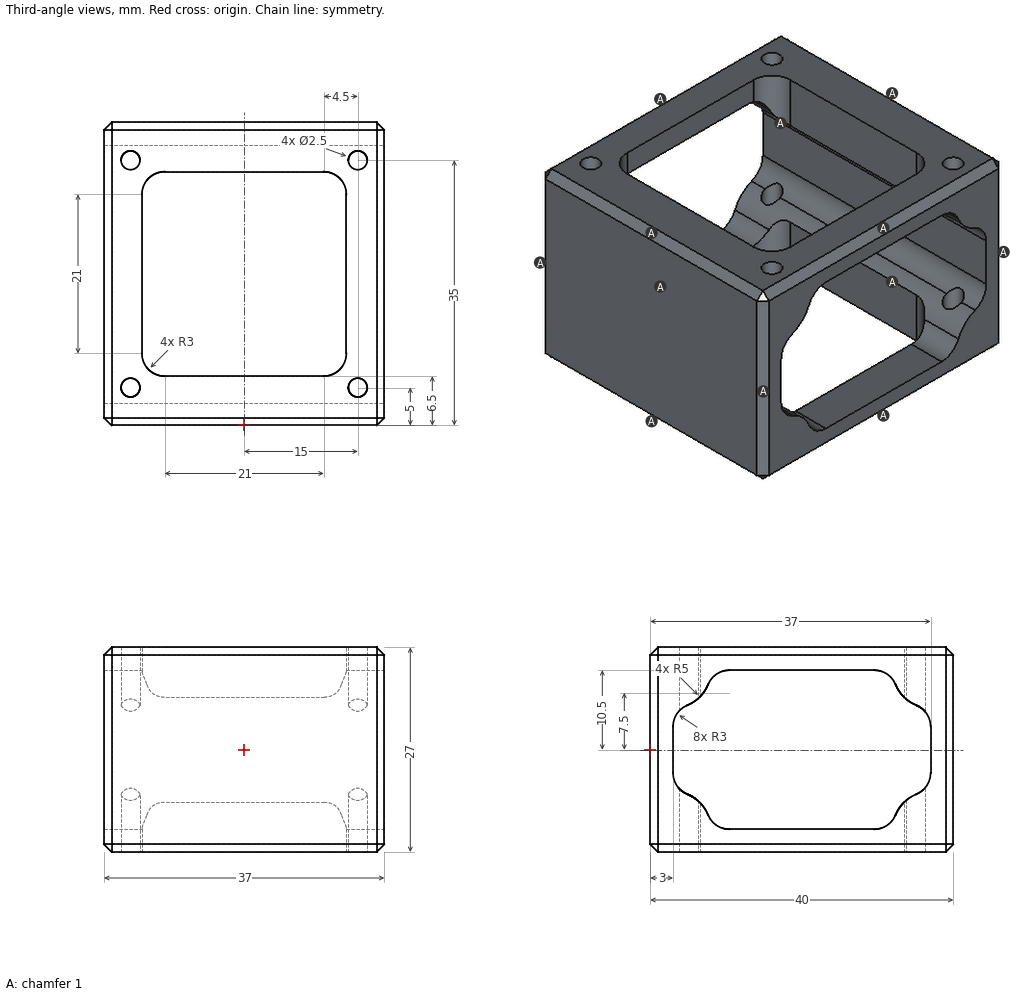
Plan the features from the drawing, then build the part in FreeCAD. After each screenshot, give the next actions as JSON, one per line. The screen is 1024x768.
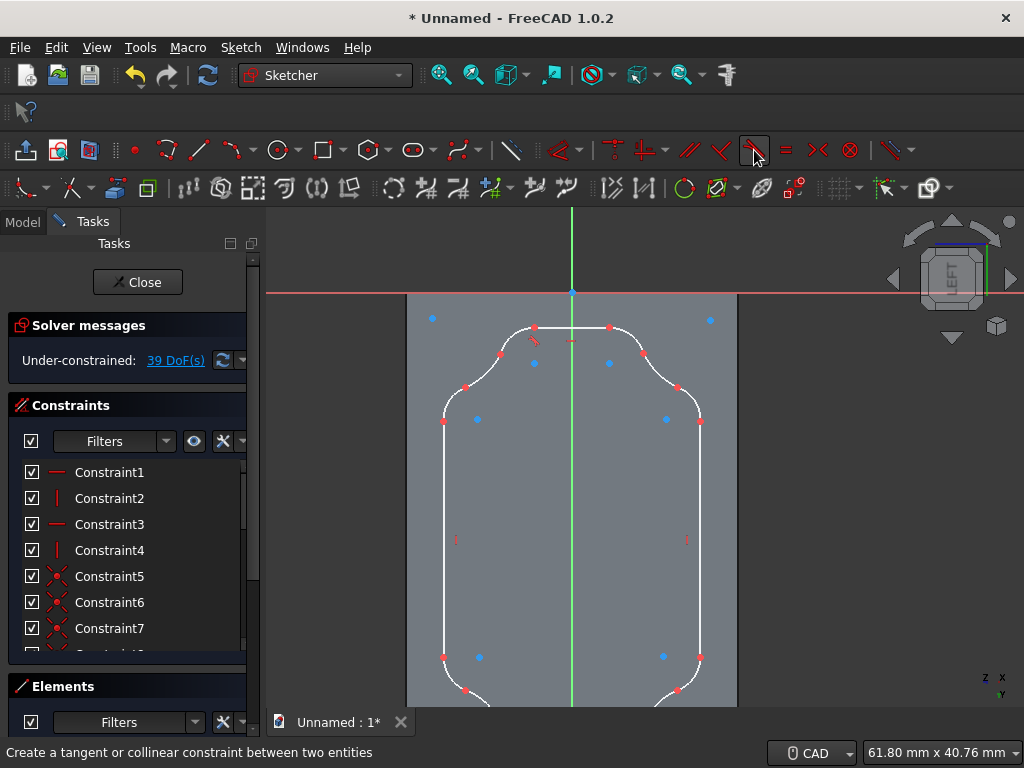
{"action": "left_click", "coordinate": [587, 328]}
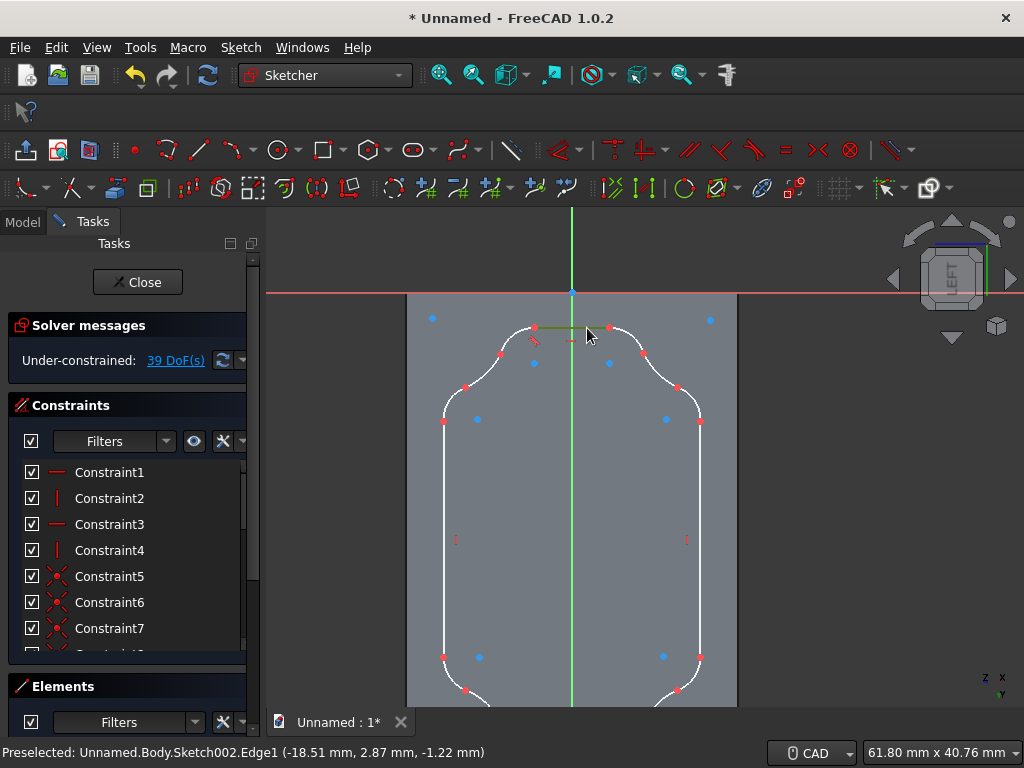
{"action": "left_click", "coordinate": [637, 341]}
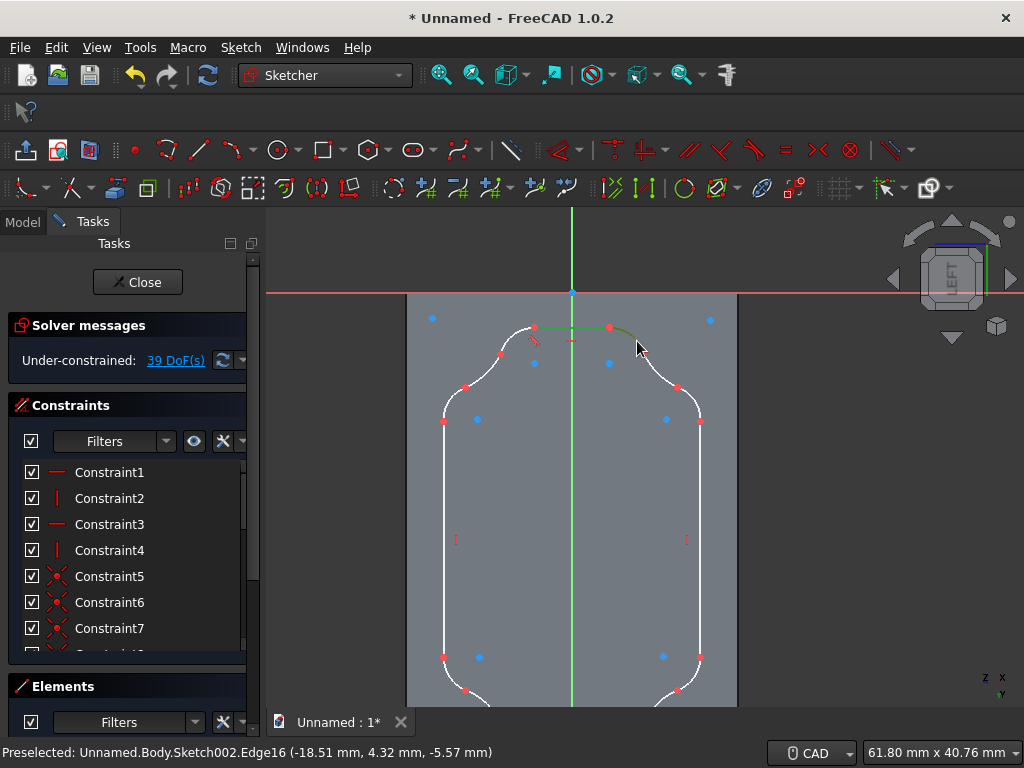
{"action": "key", "text": "t"}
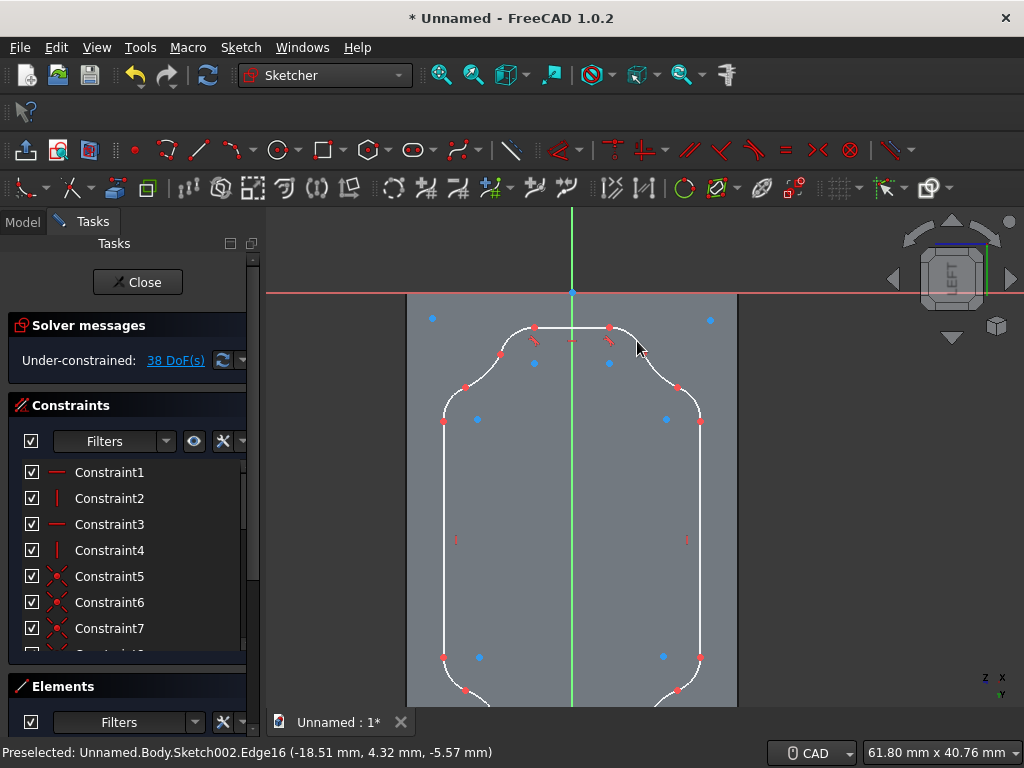
{"action": "left_click", "coordinate": [444, 492]}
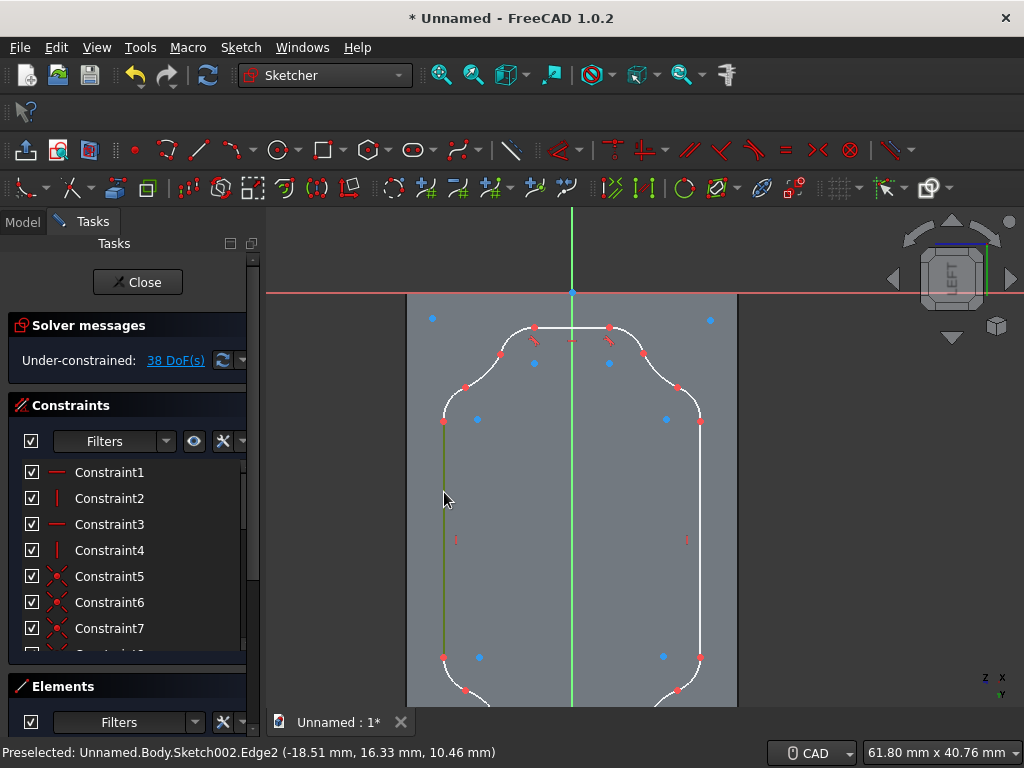
{"action": "left_click", "coordinate": [455, 394]}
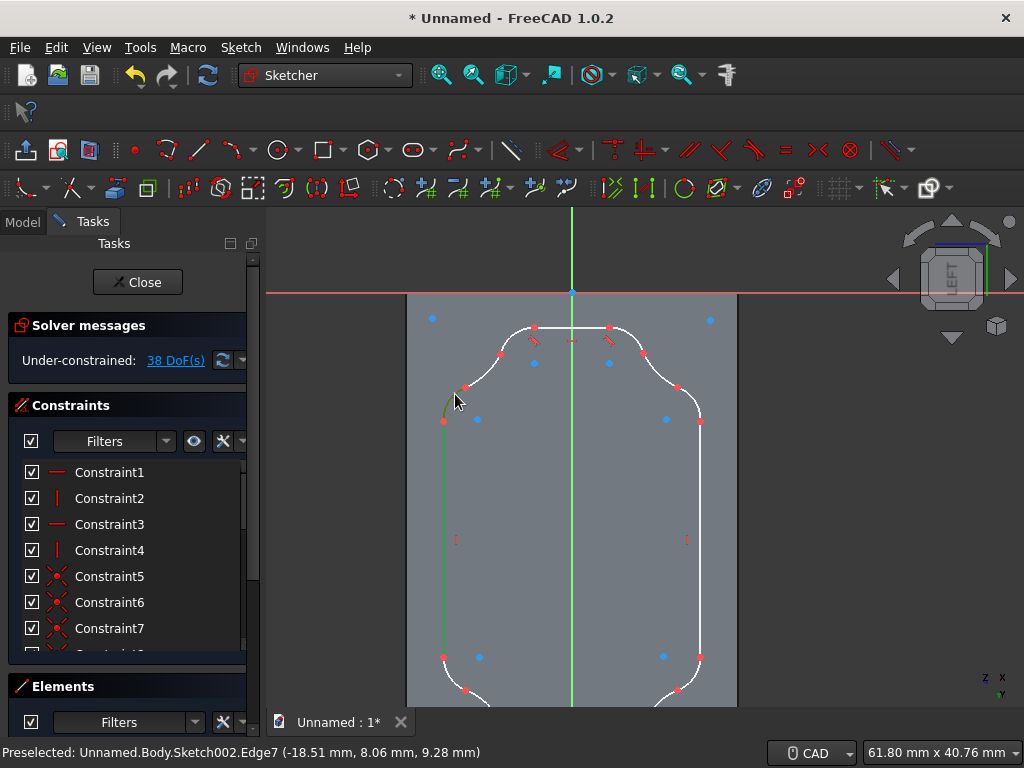
{"action": "key", "text": "t"}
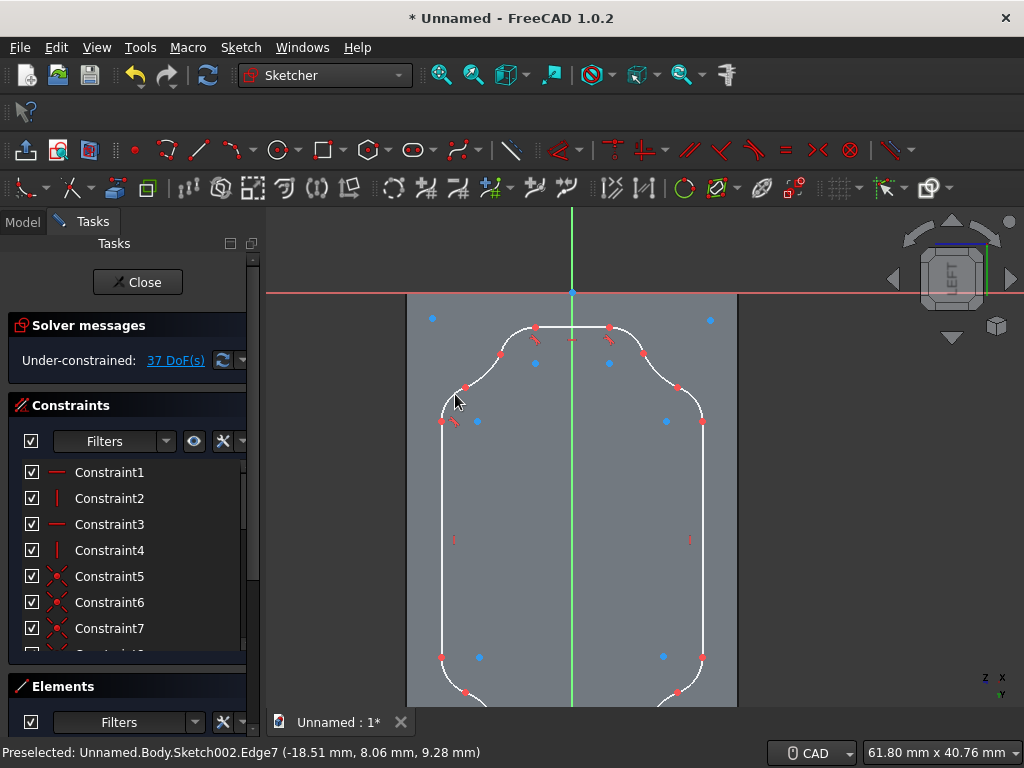
{"action": "left_click", "coordinate": [442, 492]}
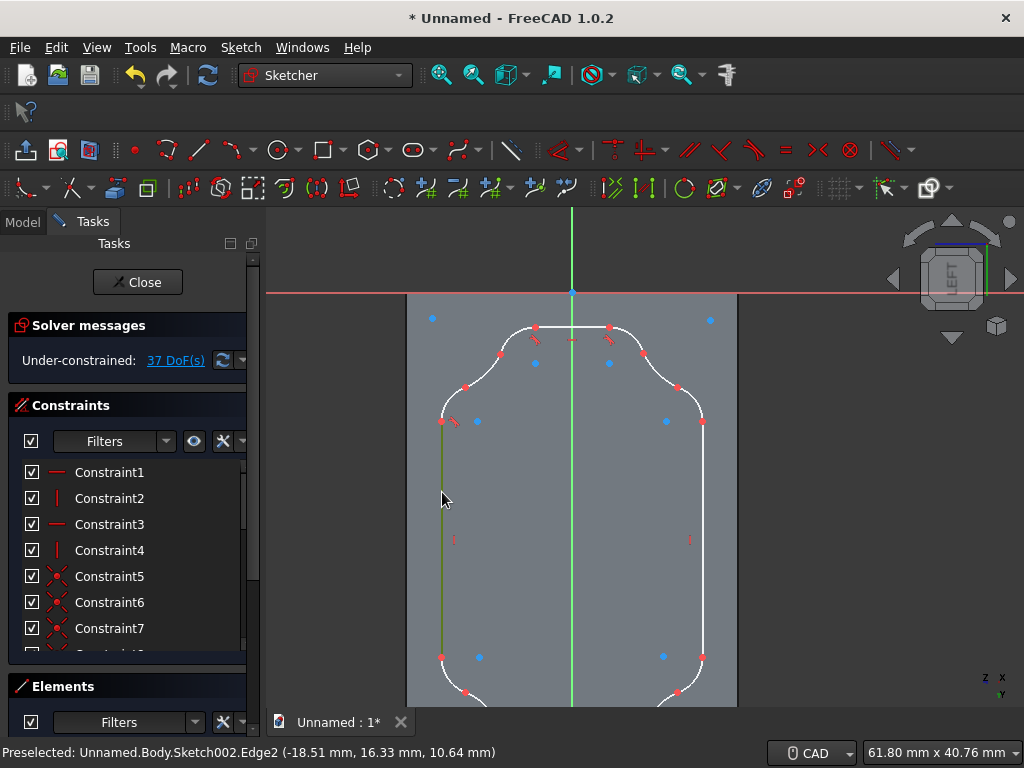
{"action": "left_click", "coordinate": [444, 671]}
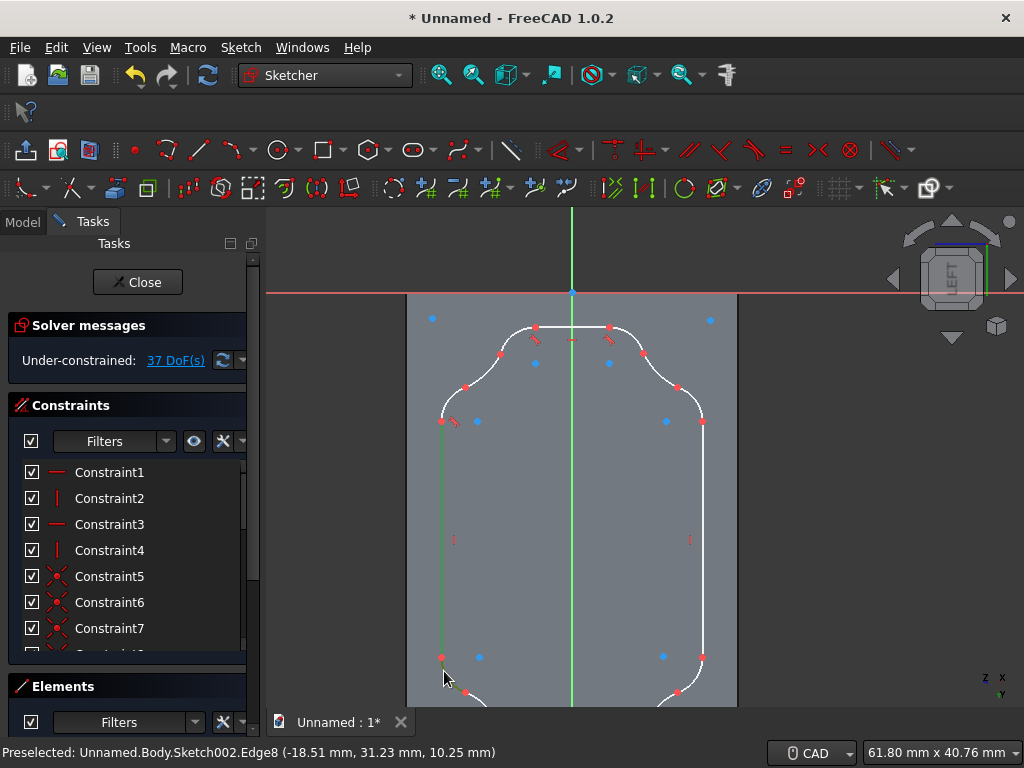
{"action": "key", "text": "t"}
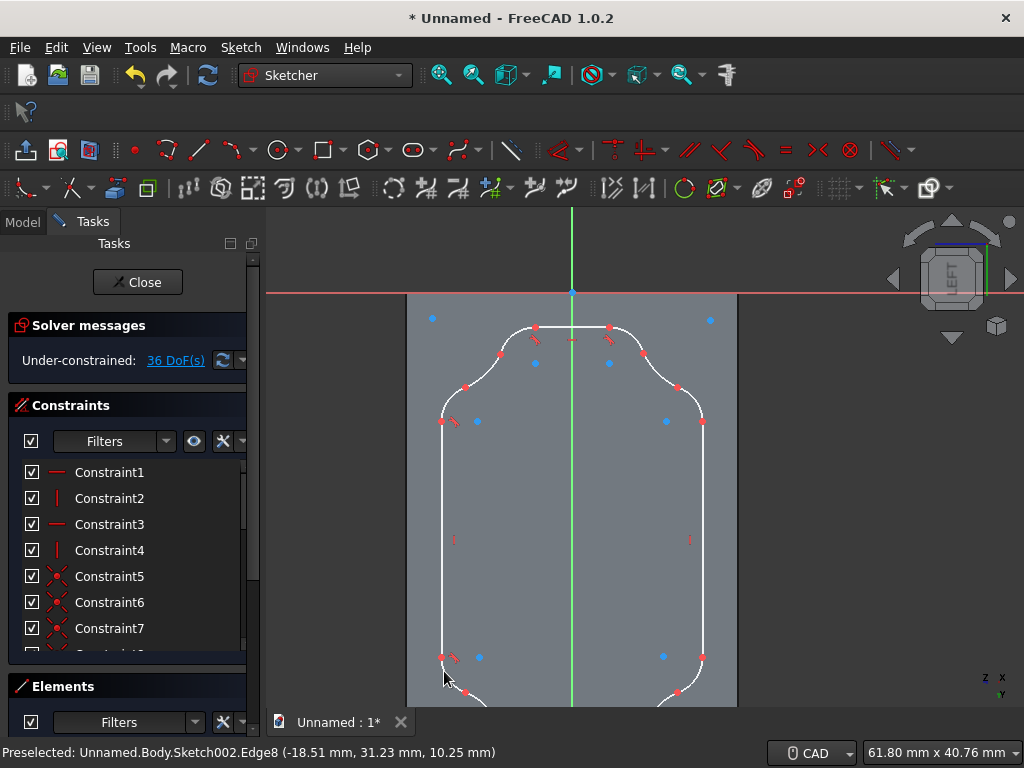
{"action": "scroll", "coordinate": [586, 330], "scroll_direction": "down", "scroll_amount": 2}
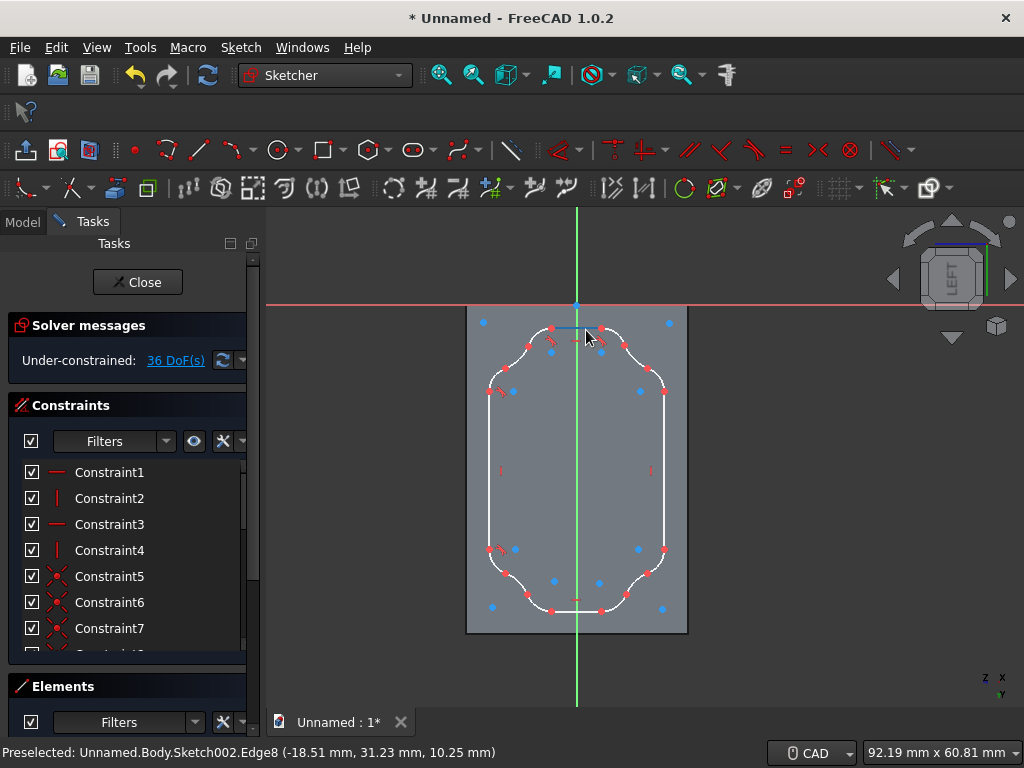
{"action": "scroll", "coordinate": [567, 612], "scroll_direction": "up", "scroll_amount": 2}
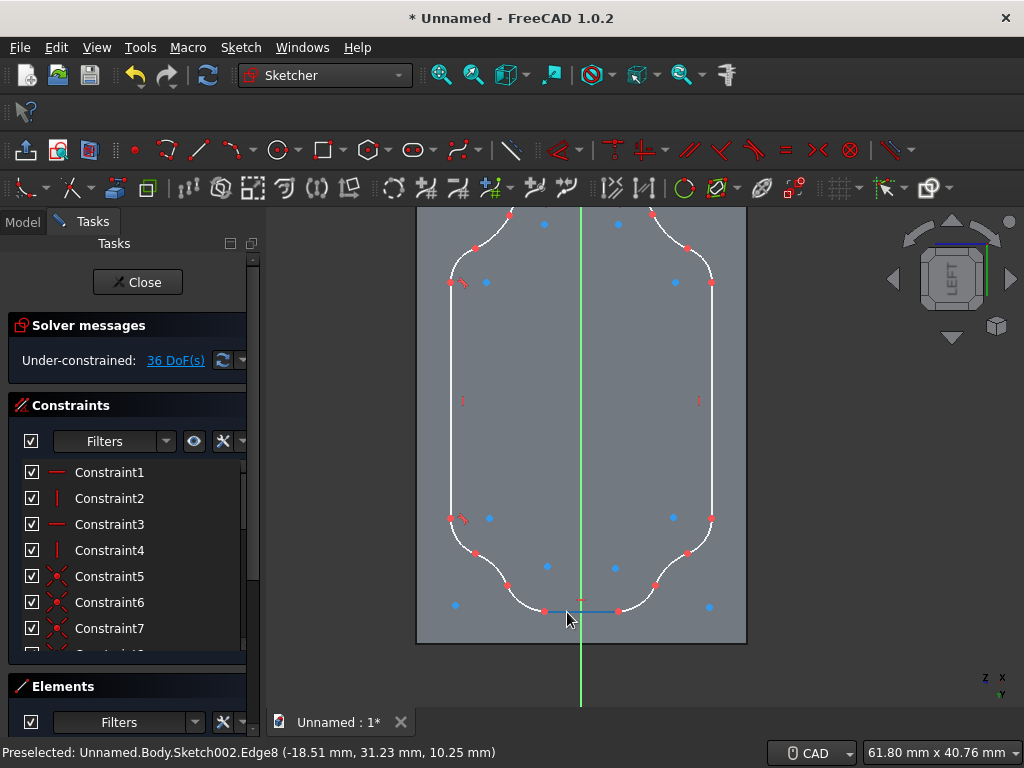
{"action": "left_click", "coordinate": [566, 612]}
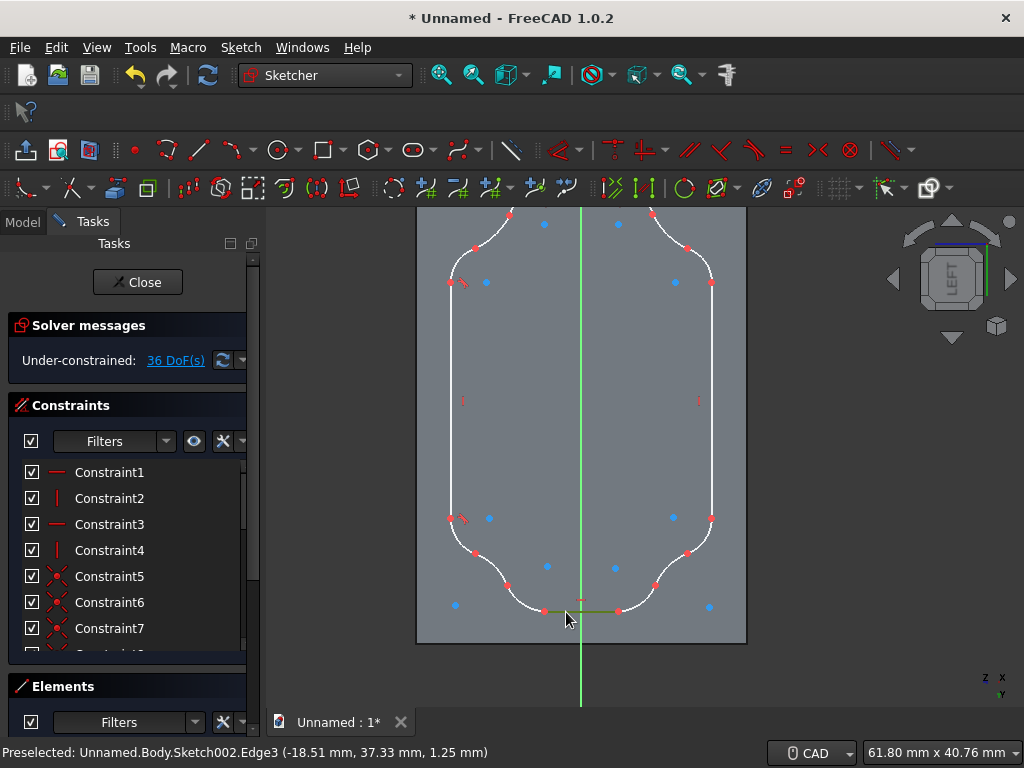
{"action": "left_click", "coordinate": [515, 597]}